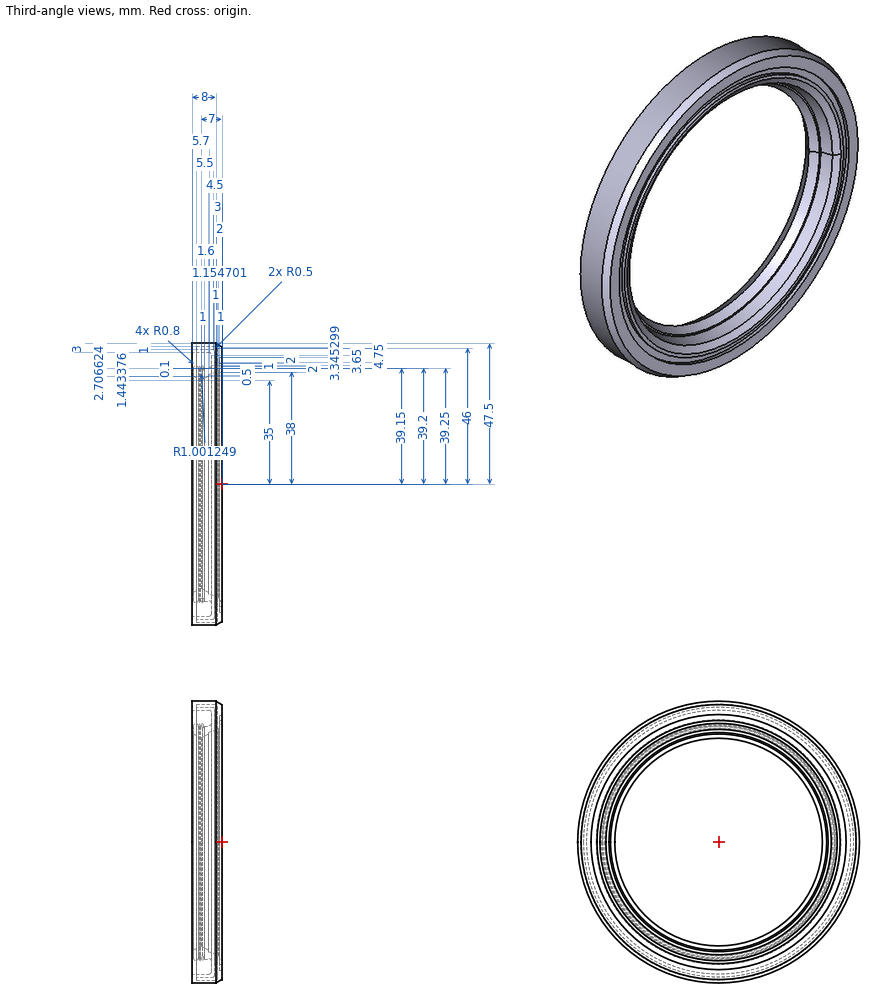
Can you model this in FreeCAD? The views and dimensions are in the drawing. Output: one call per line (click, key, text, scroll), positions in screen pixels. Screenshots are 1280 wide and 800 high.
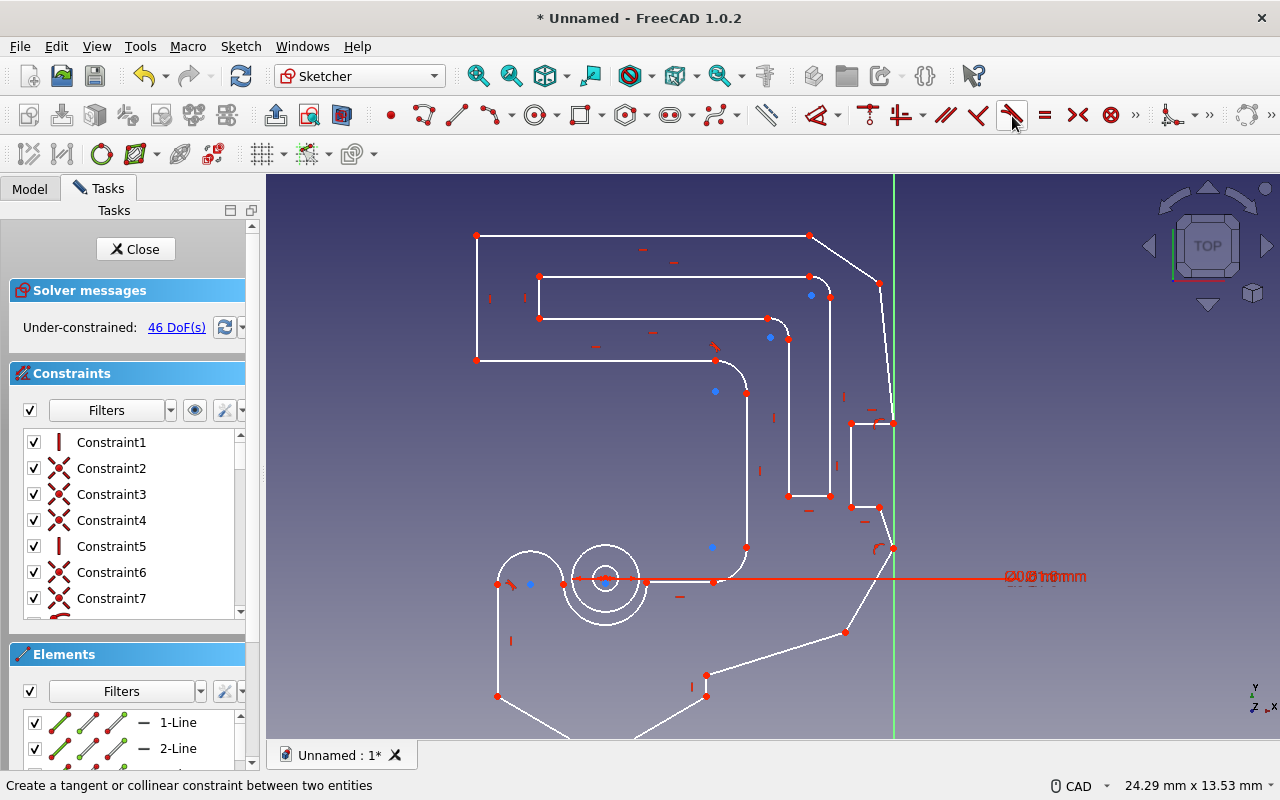
click(747, 440)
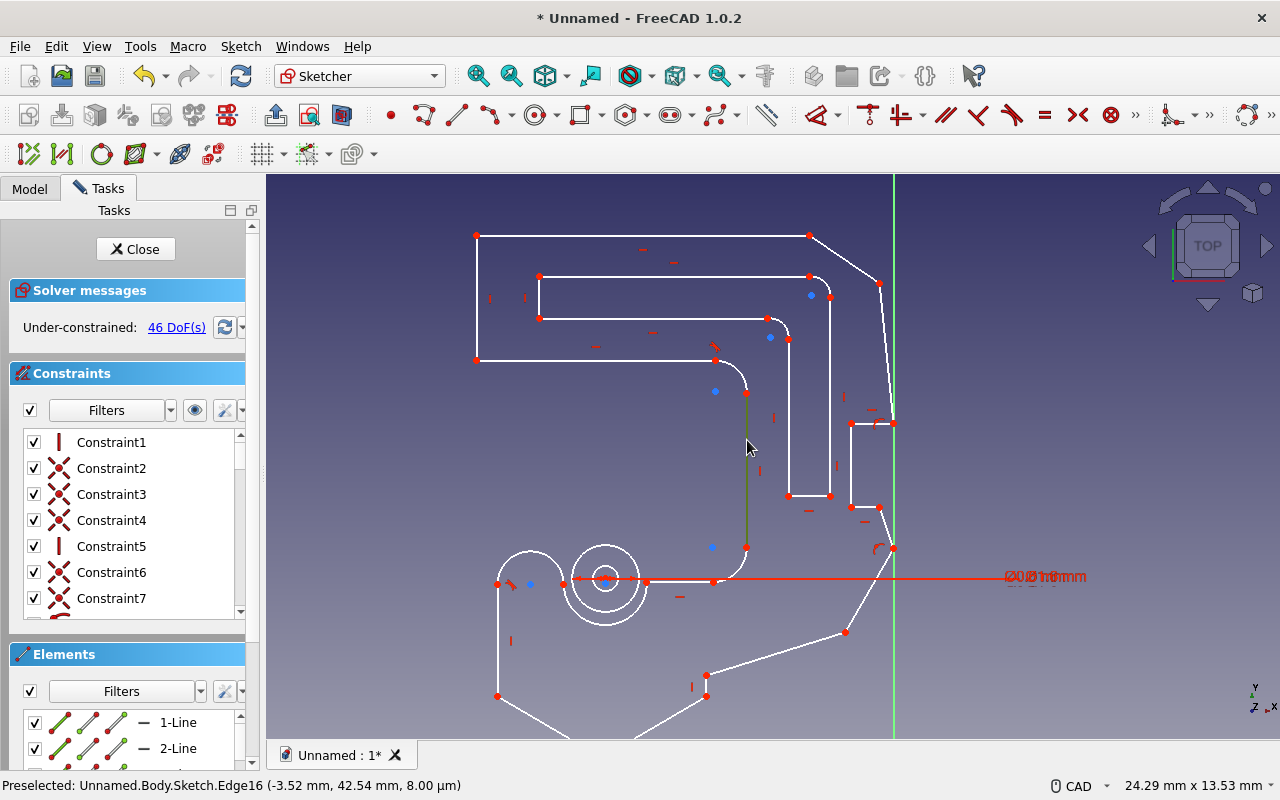
click(744, 379)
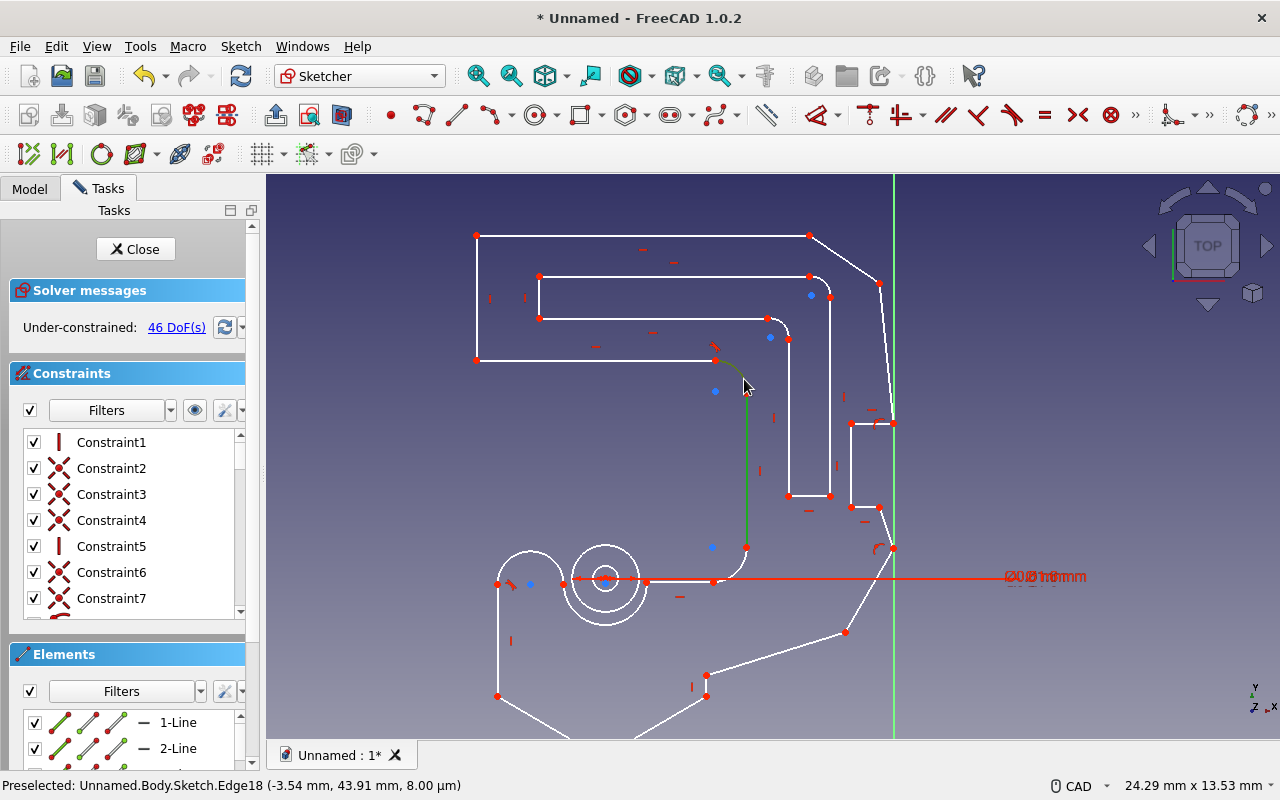
click(1012, 116)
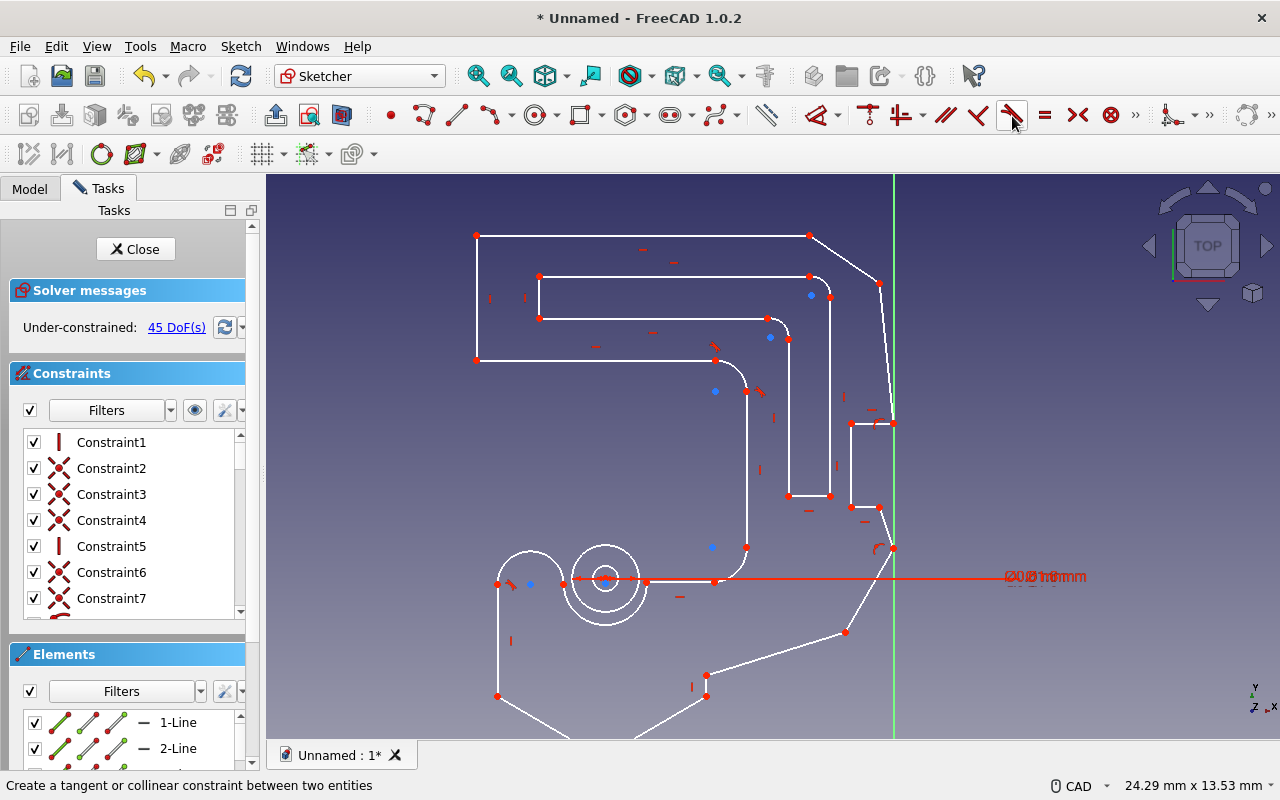
click(747, 438)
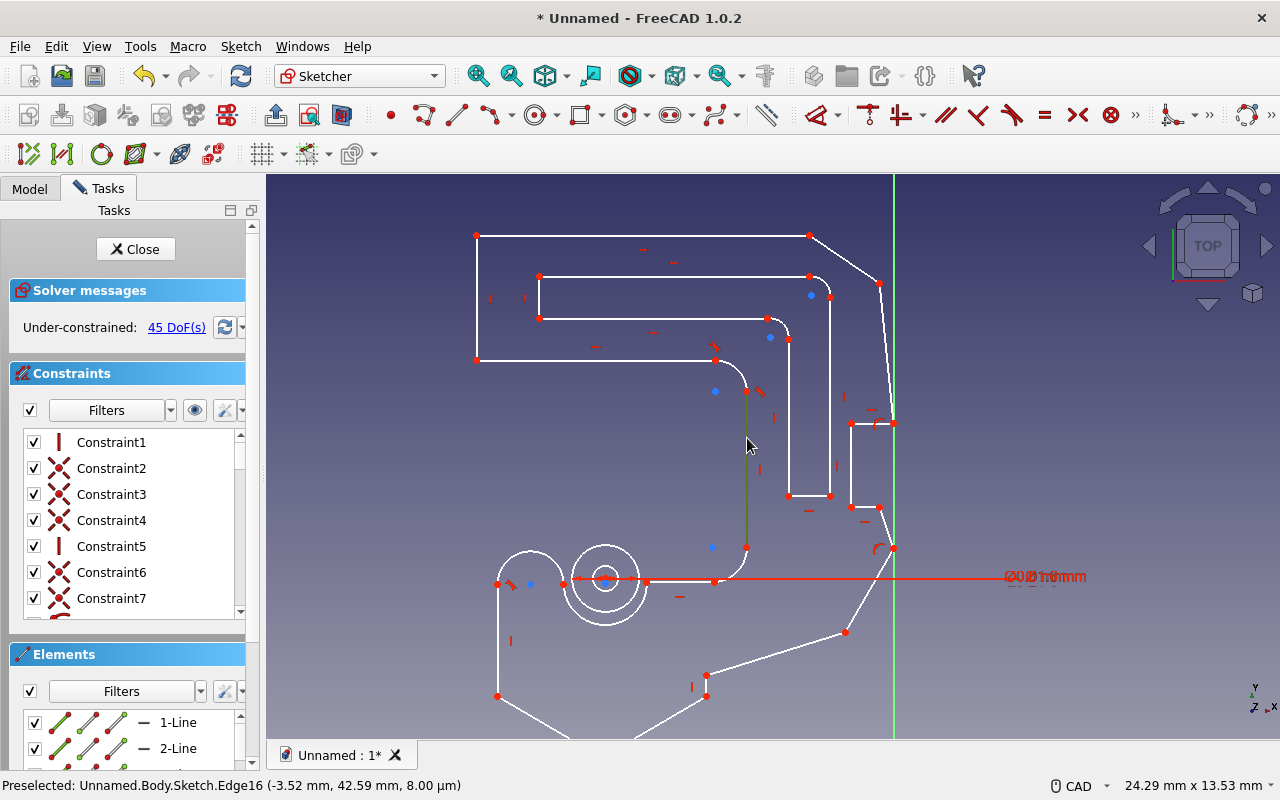
click(729, 578)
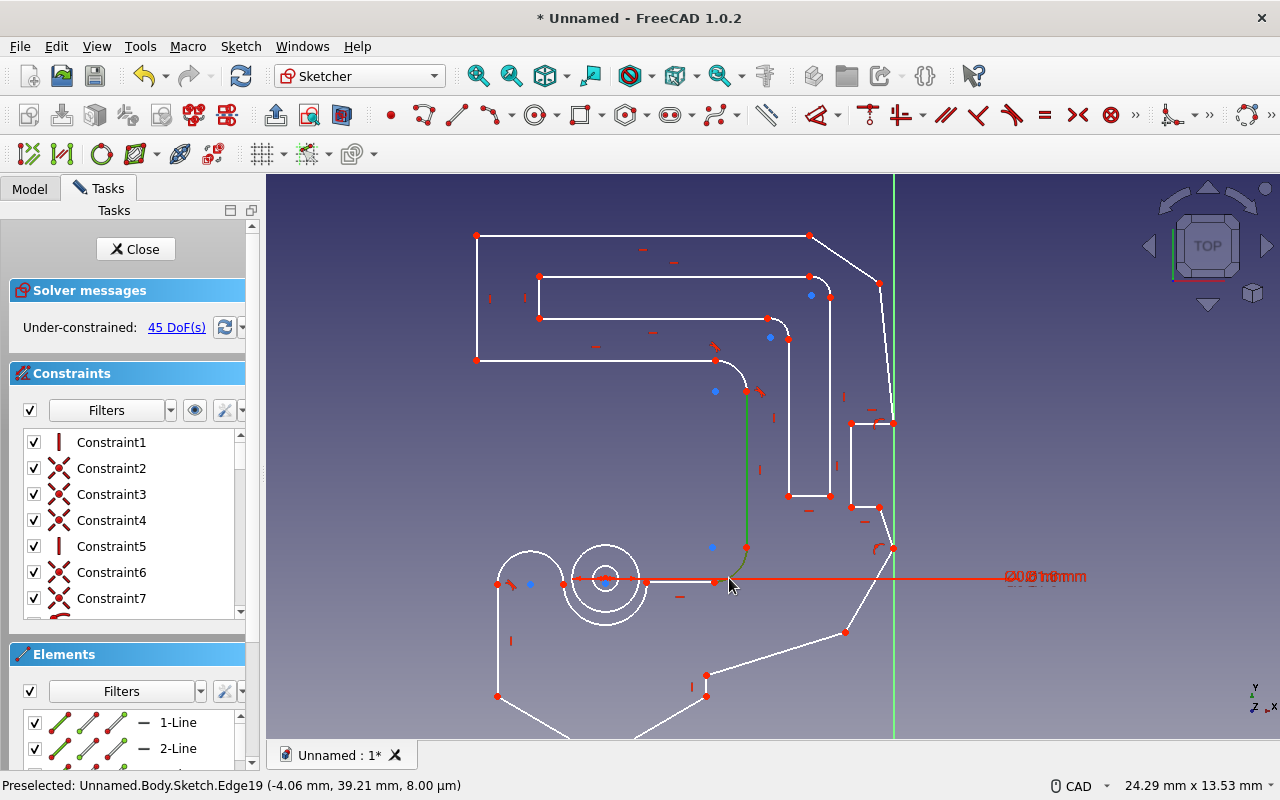
click(1012, 116)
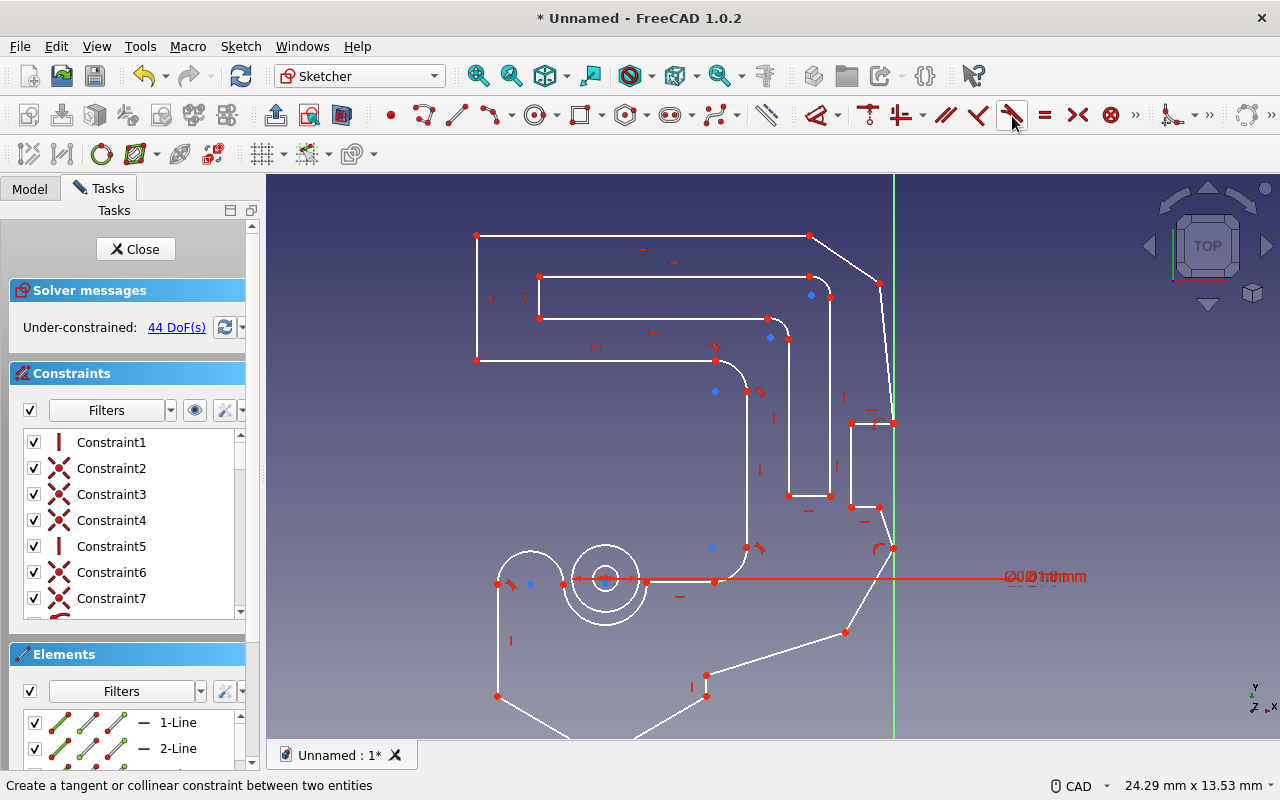
click(694, 582)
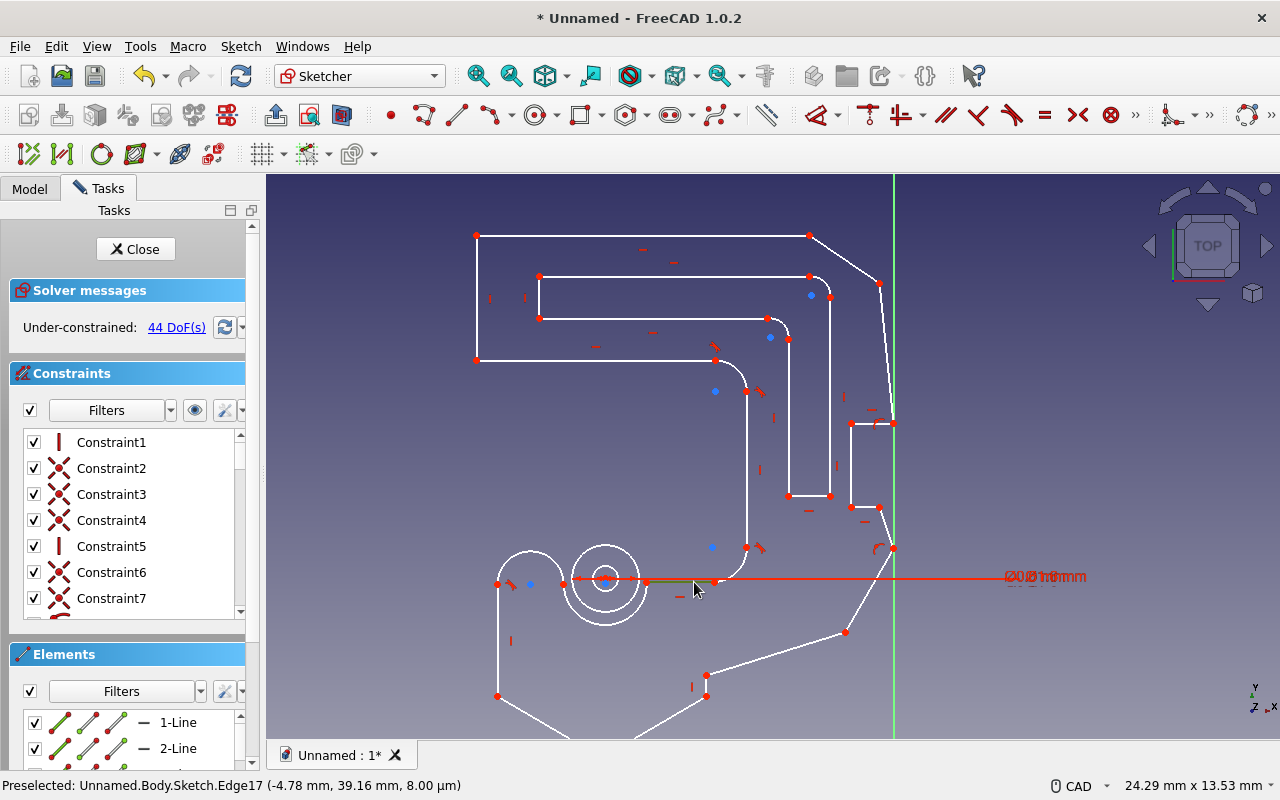
click(729, 578)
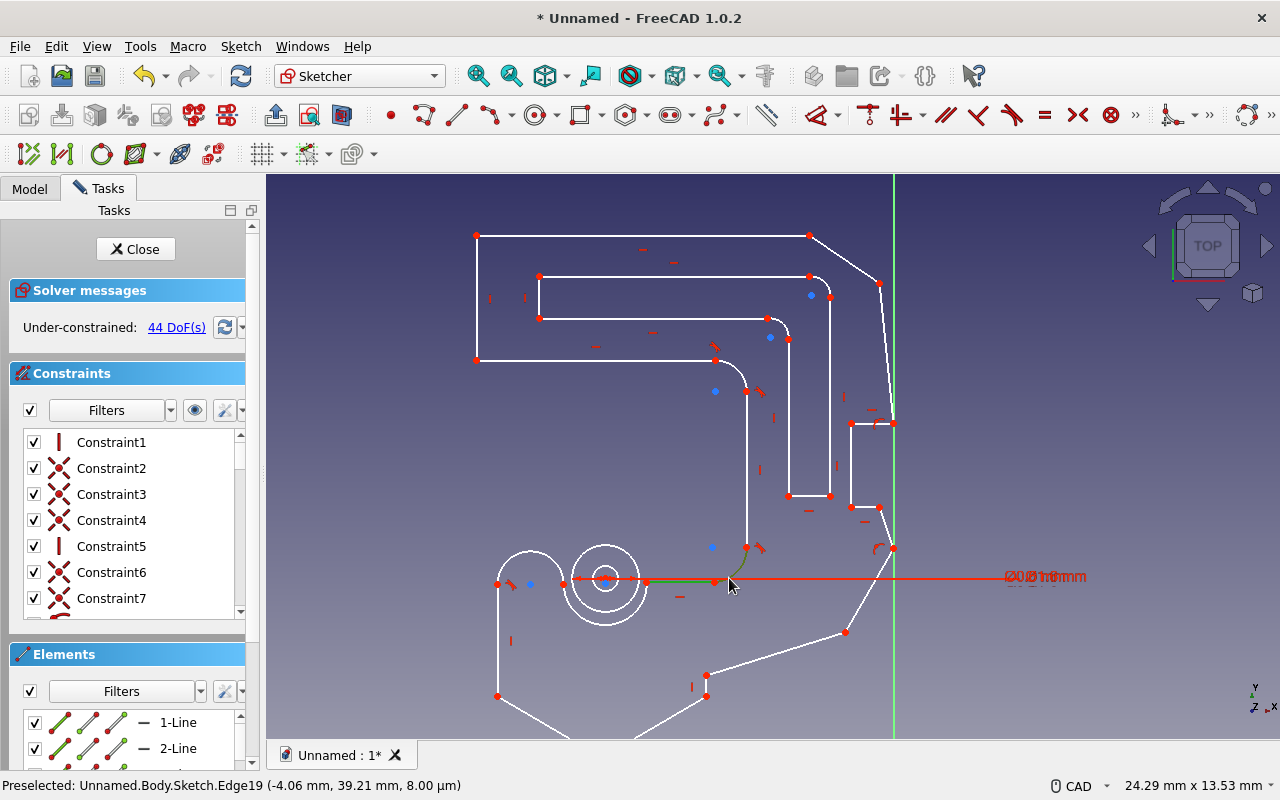
click(1012, 116)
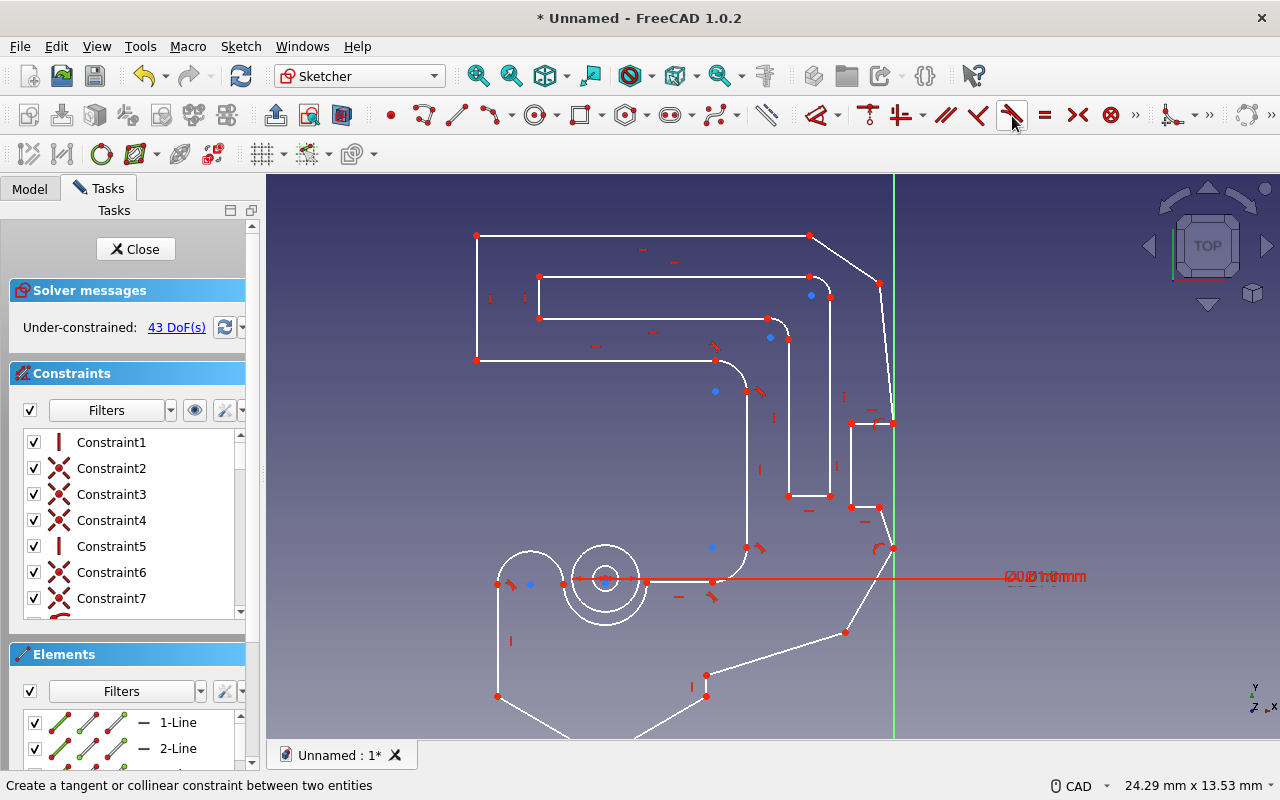
click(699, 319)